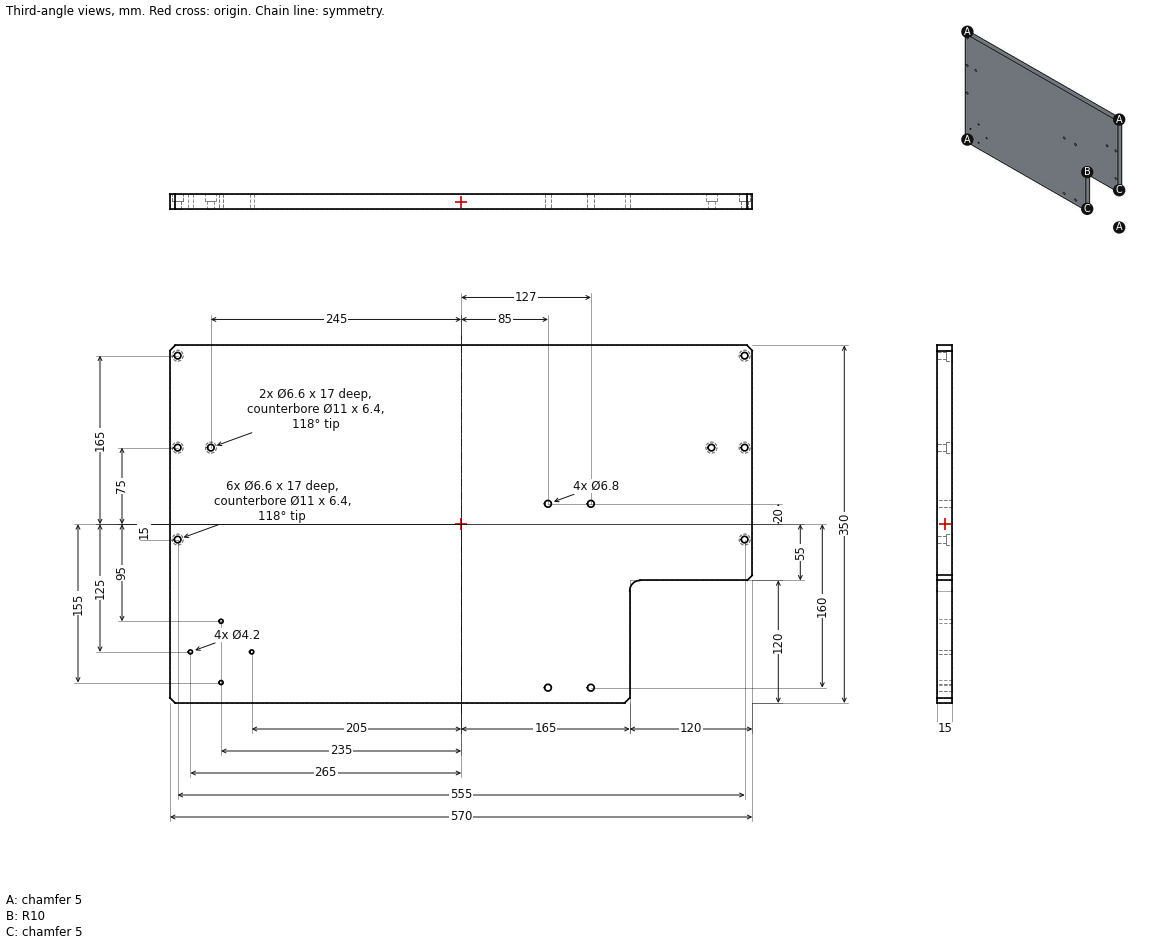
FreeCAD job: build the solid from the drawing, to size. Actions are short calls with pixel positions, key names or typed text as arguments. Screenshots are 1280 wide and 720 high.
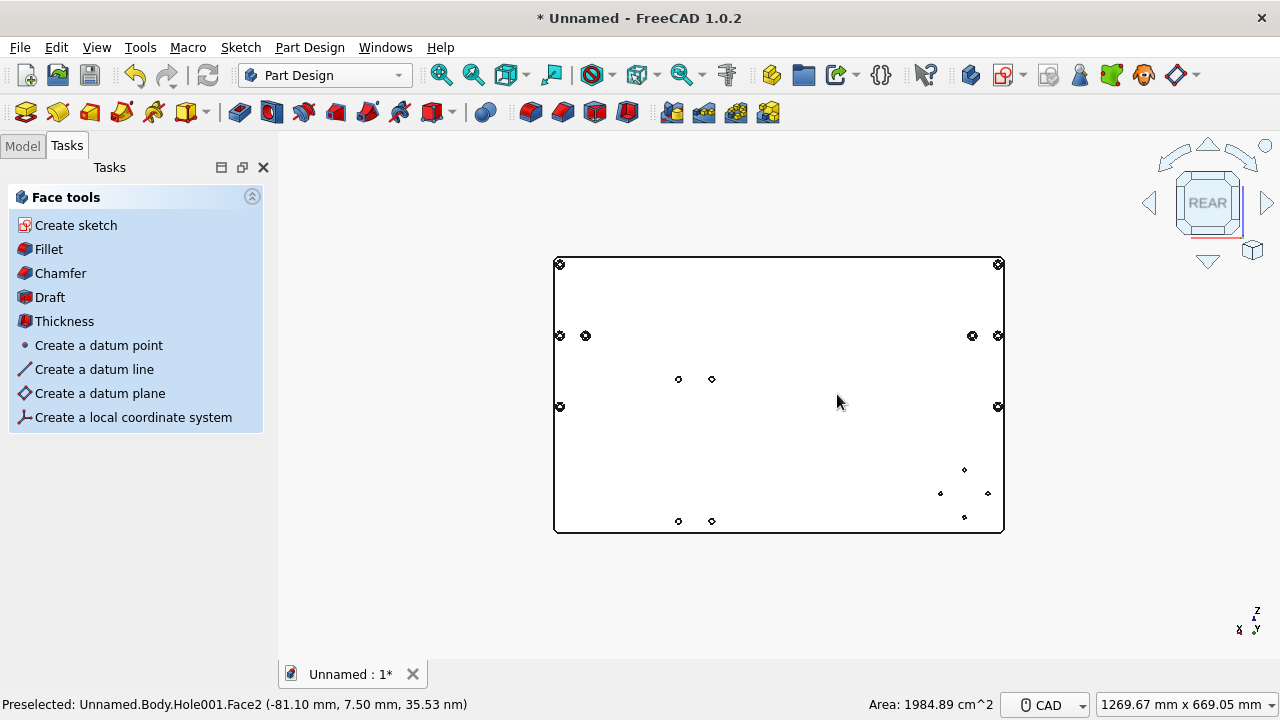
click(1004, 76)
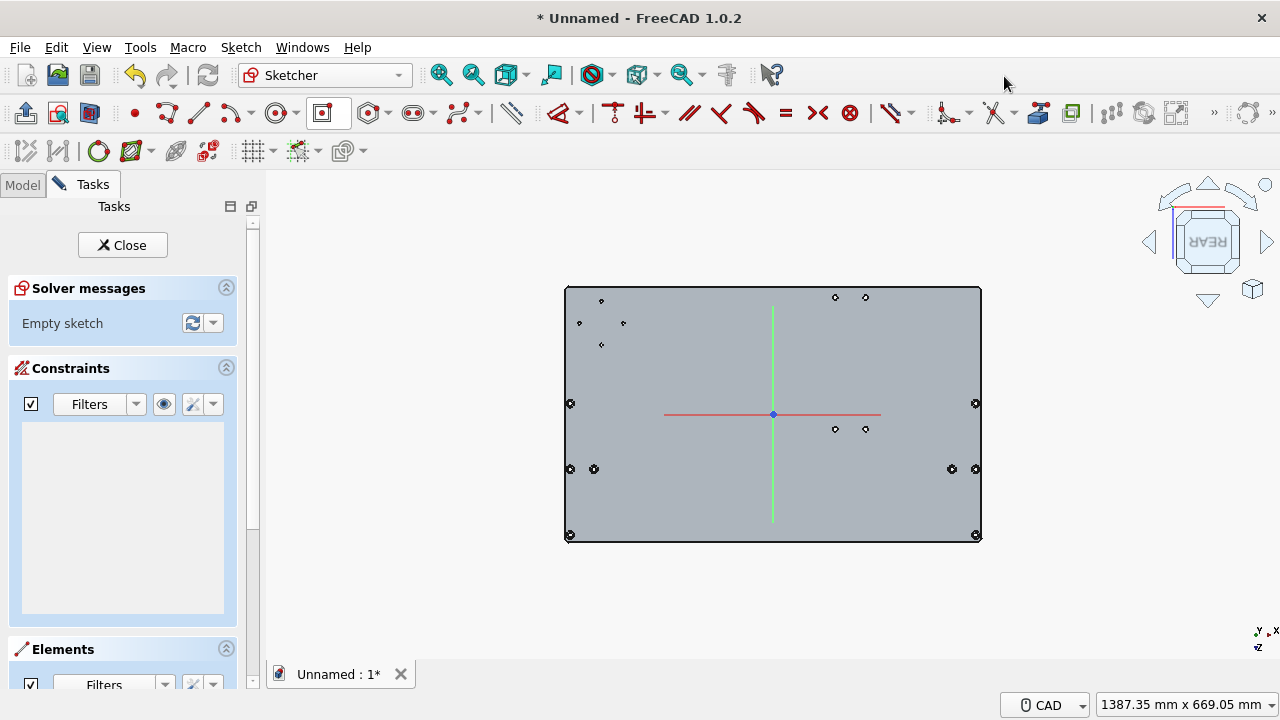
scroll(1018, 298, up, 4)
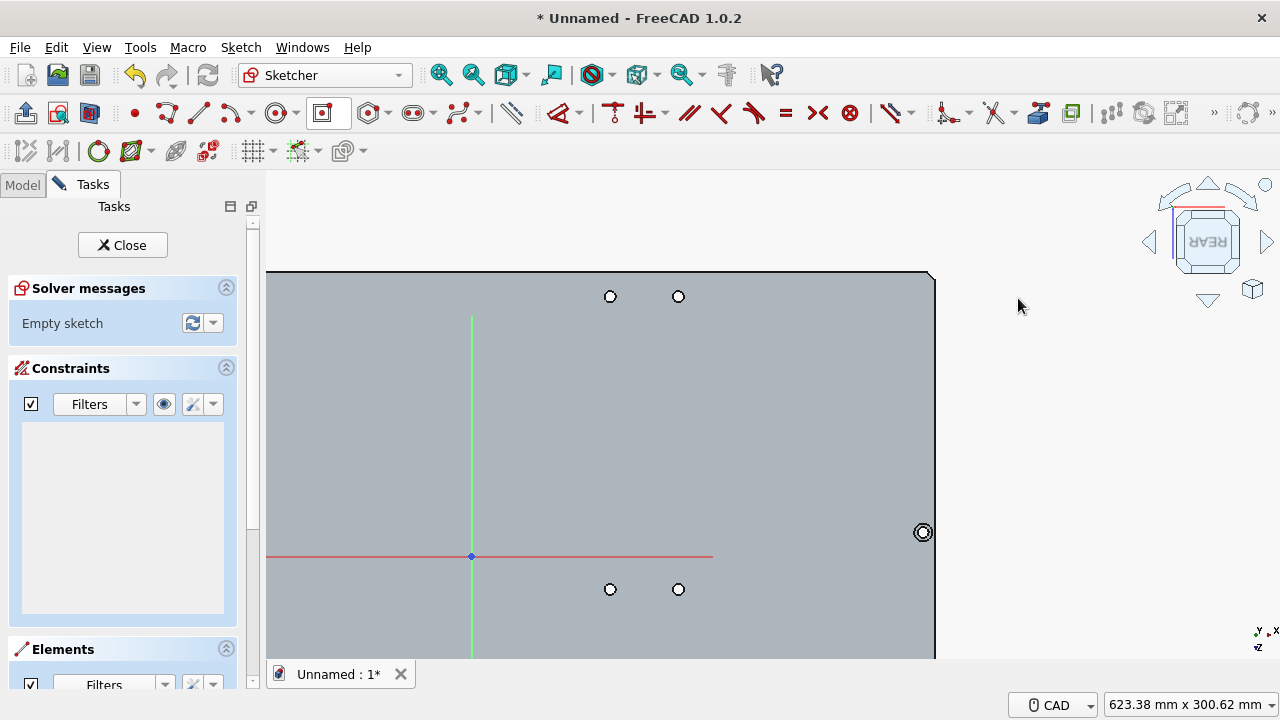
key(g)
key(r)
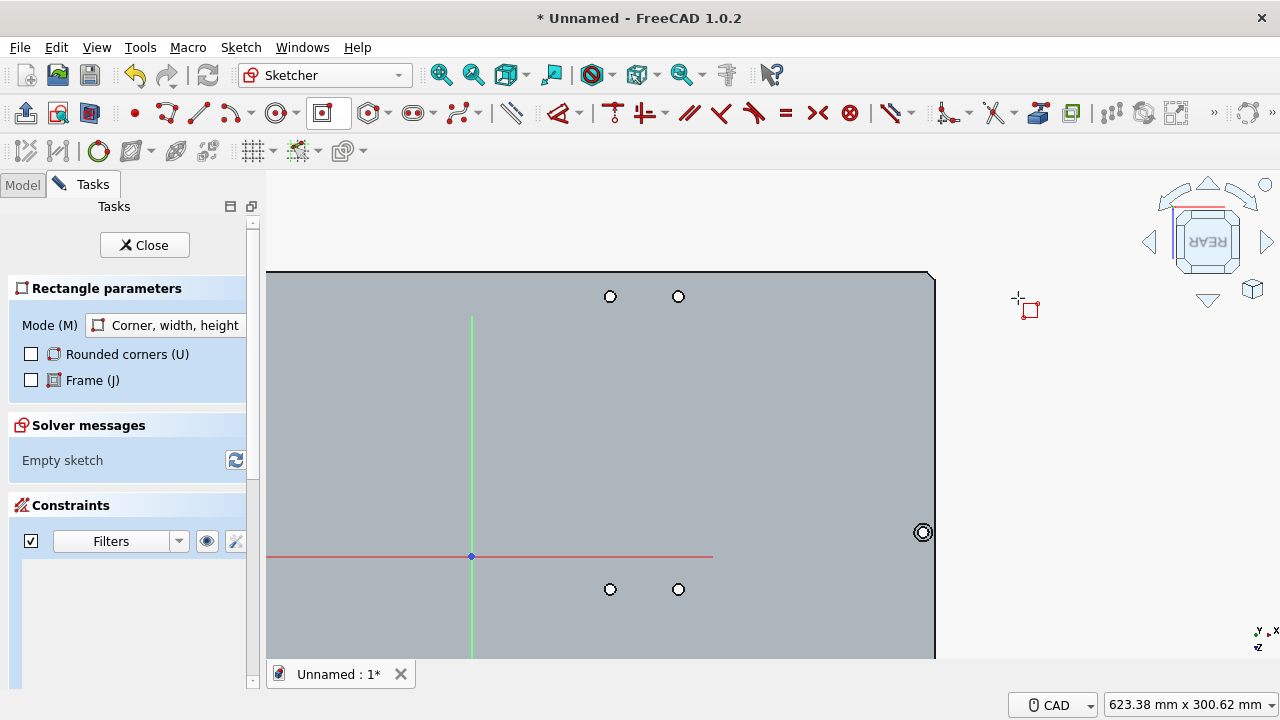
click(740, 272)
move(935, 467)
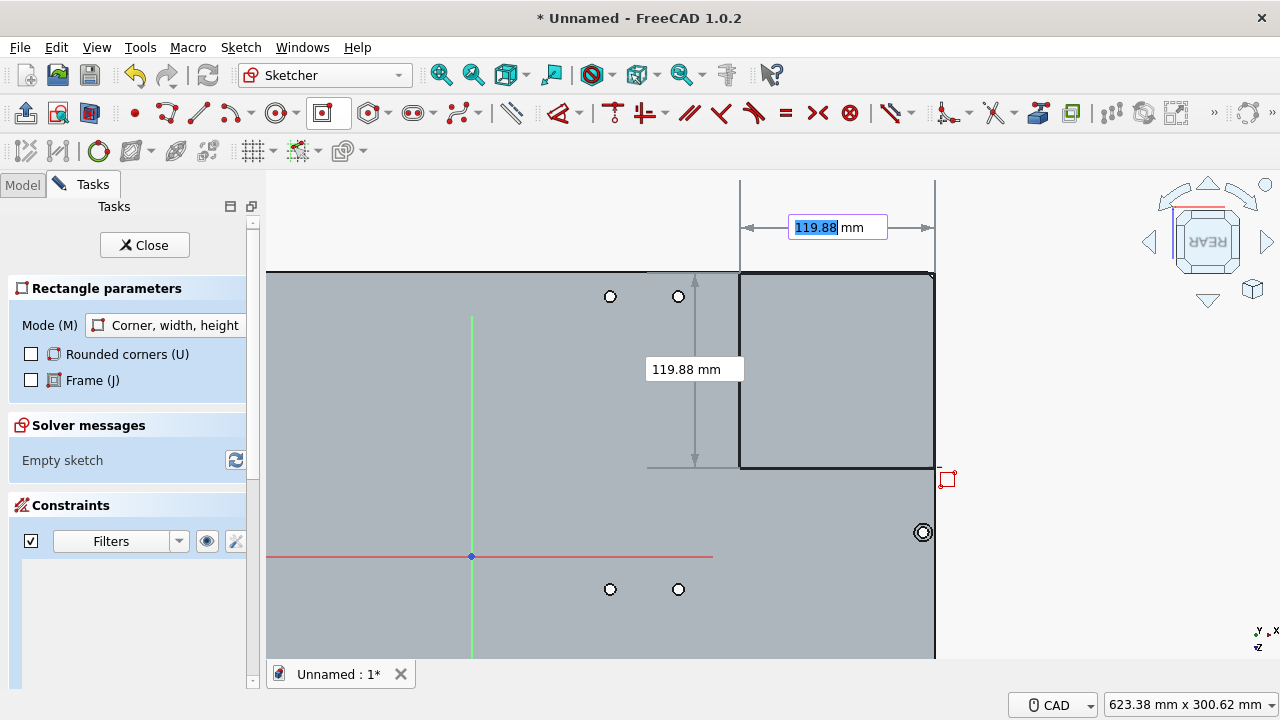
text(120)
key(Tab)
text(120)
key(Return)
key(Escape)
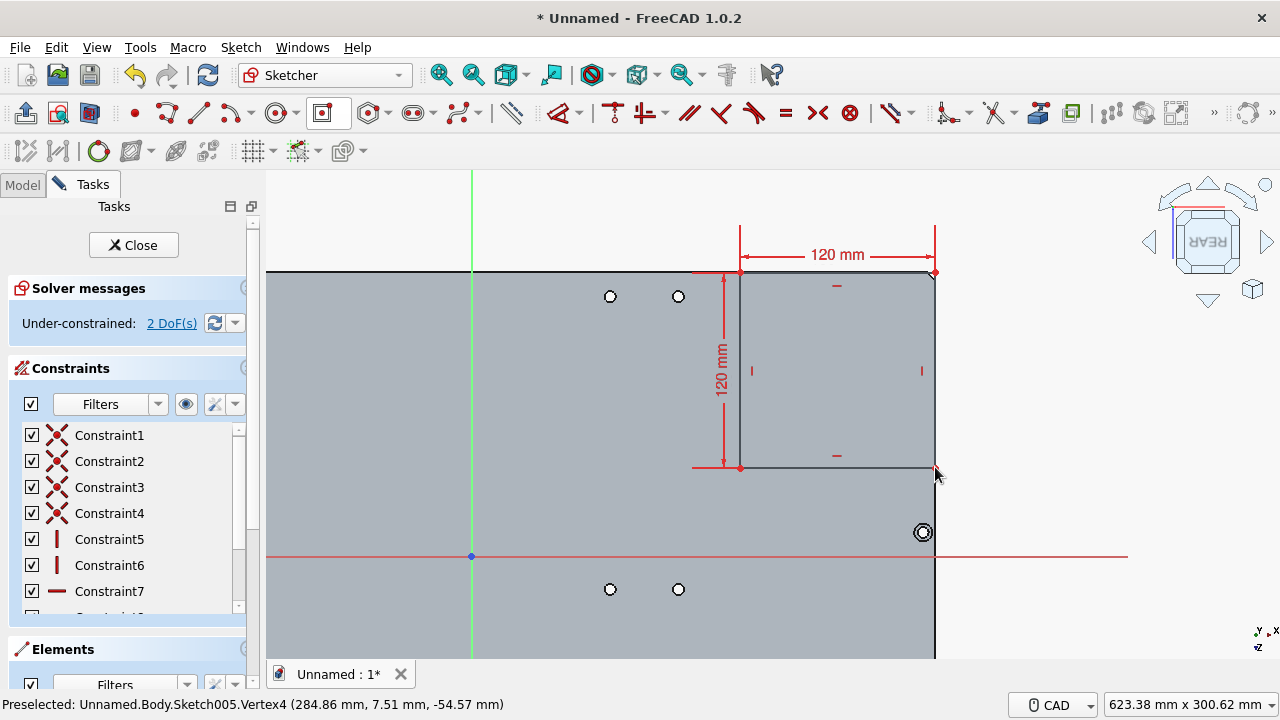
click(558, 114)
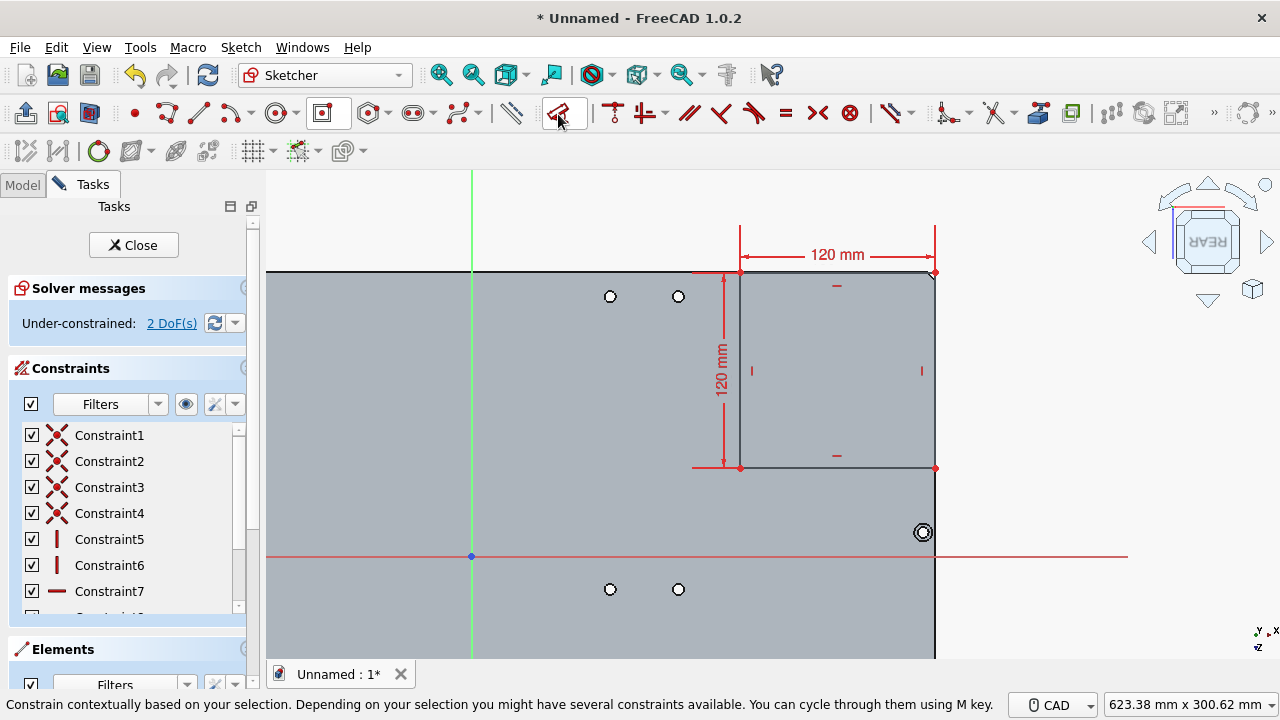
click(740, 468)
click(438, 513)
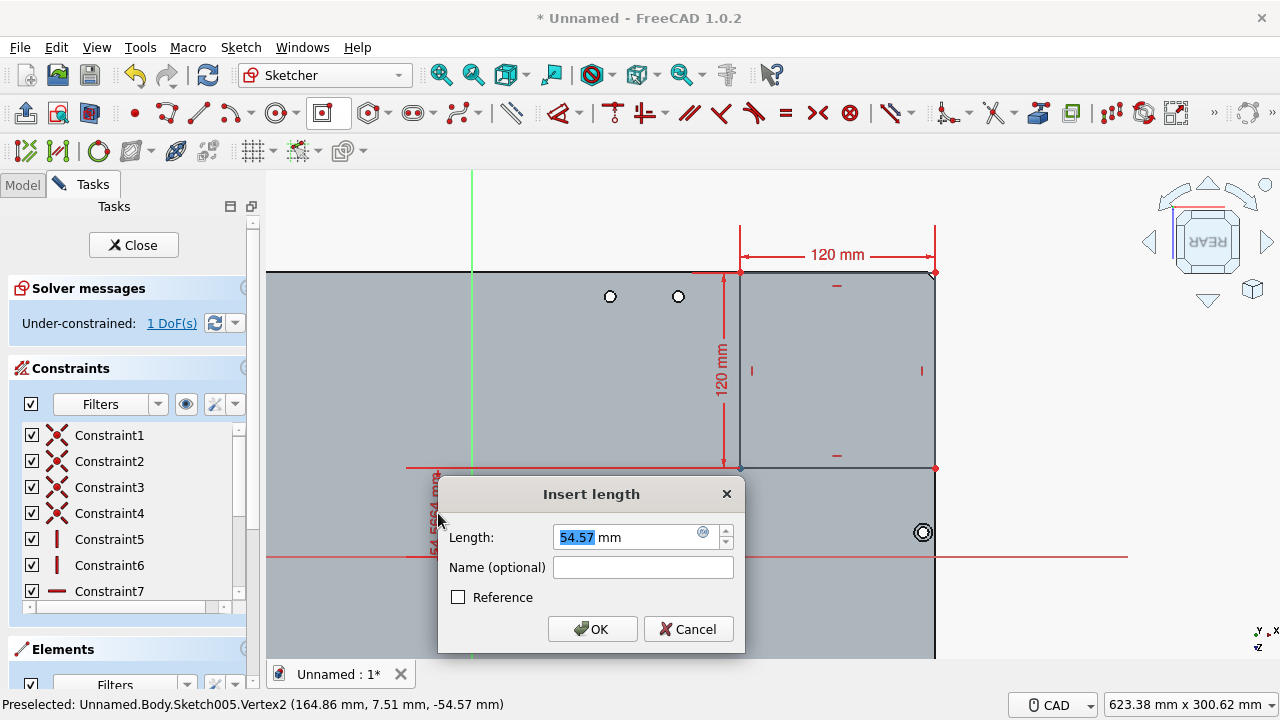
text(55)
key(Return)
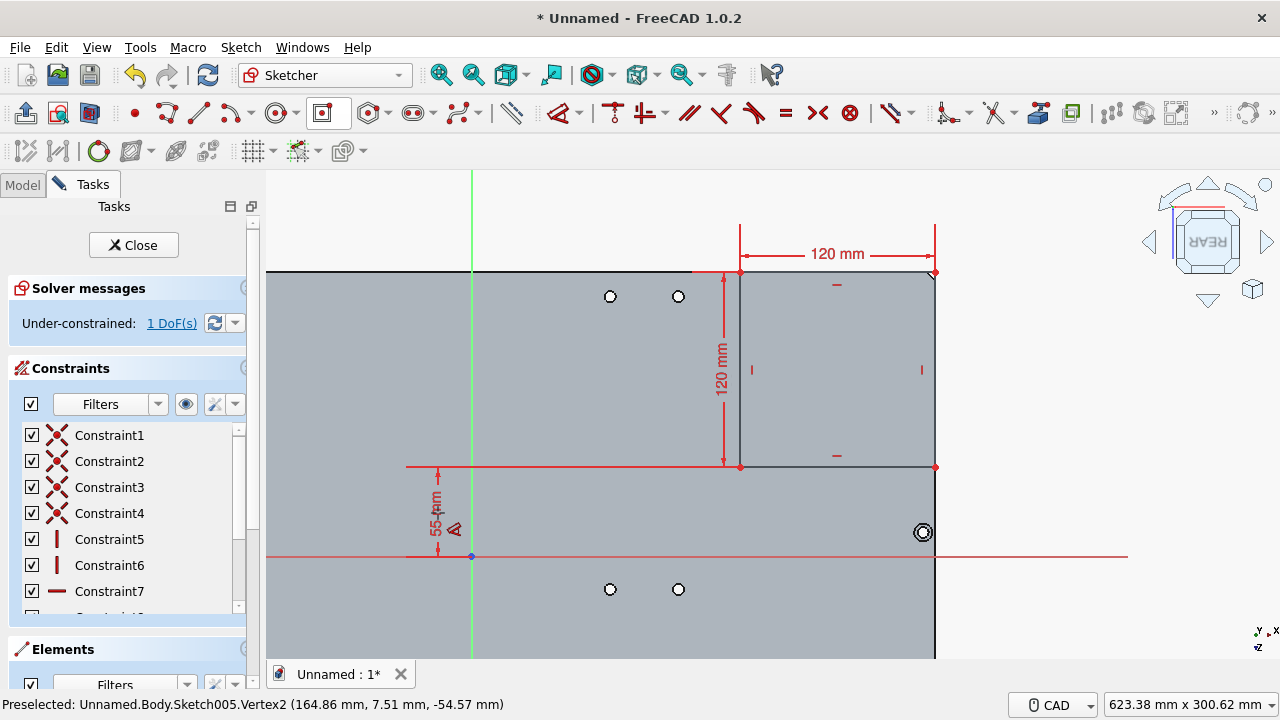
click(740, 272)
click(606, 591)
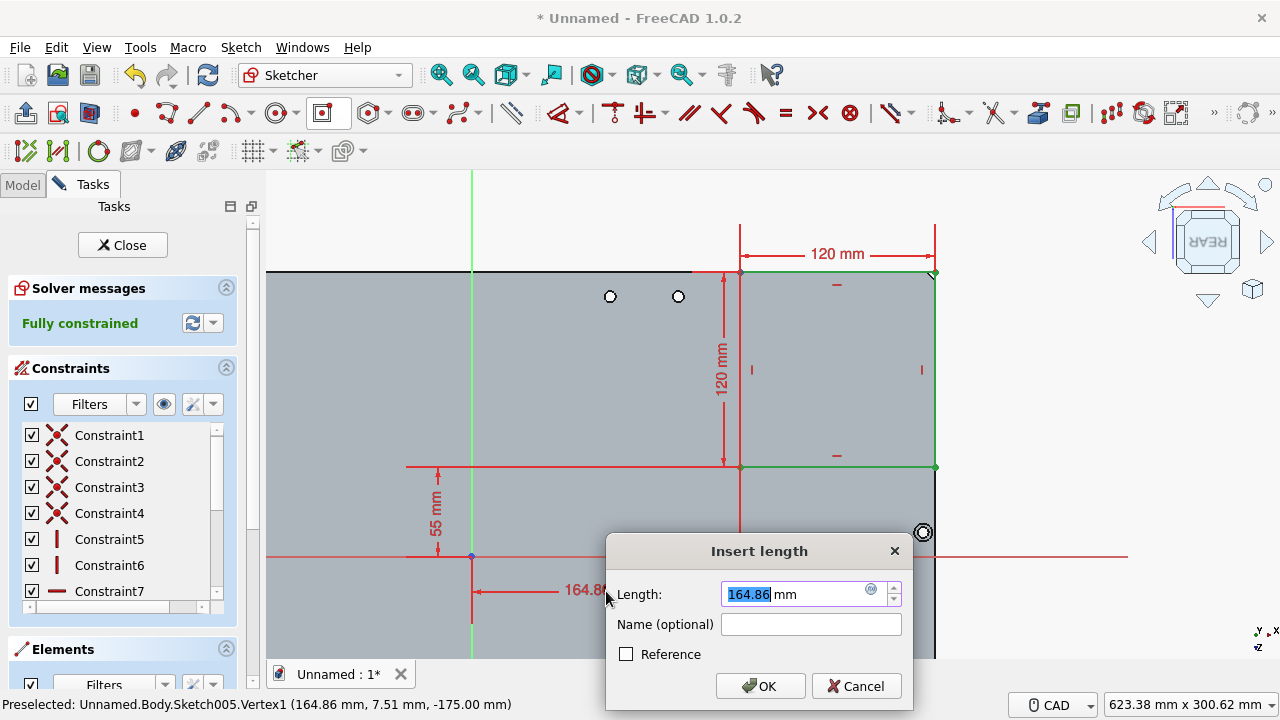
text(165)
key(Return)
key(Escape)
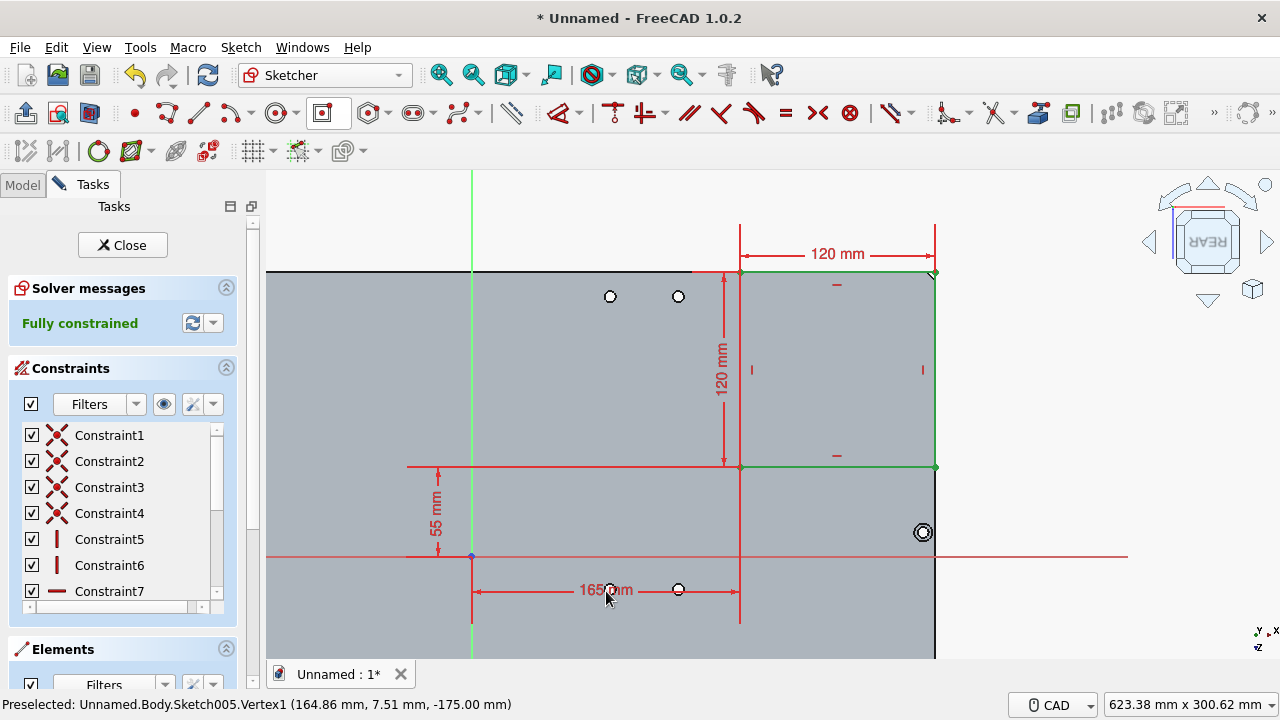
click(123, 245)